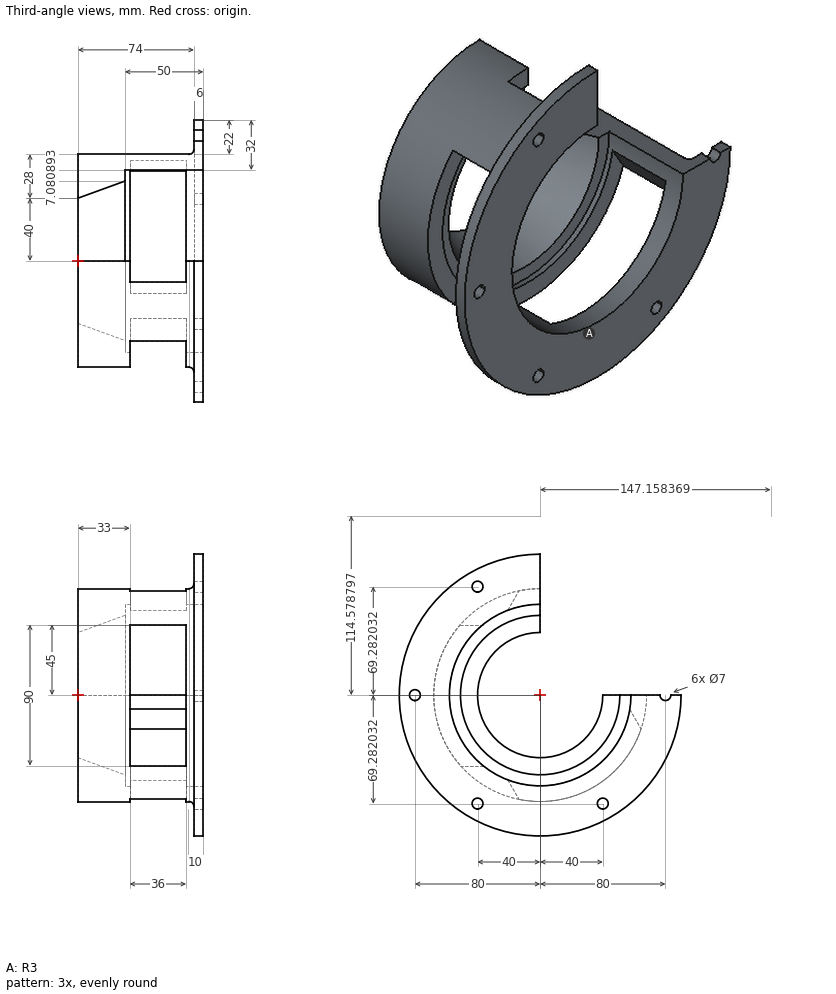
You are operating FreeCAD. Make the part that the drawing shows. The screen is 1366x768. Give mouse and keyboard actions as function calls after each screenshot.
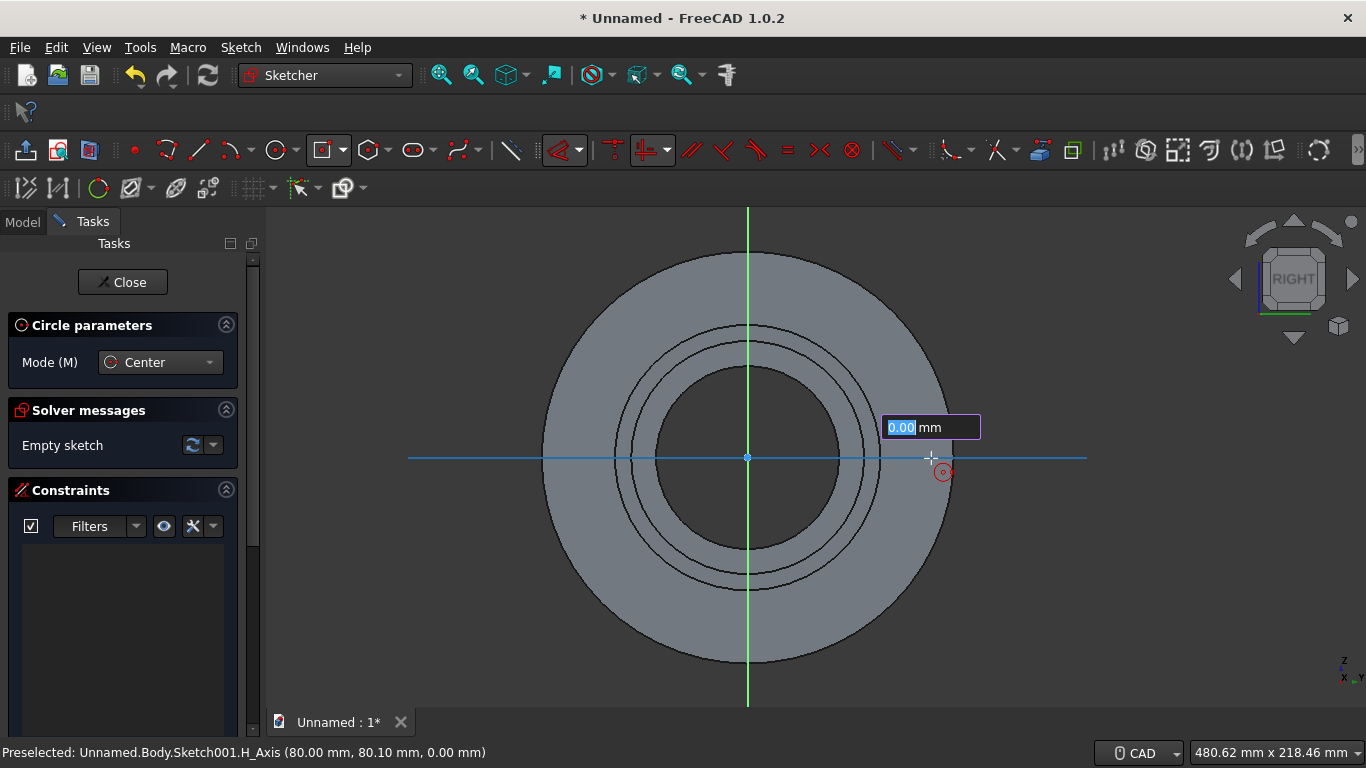
scroll(934, 450, up, 4)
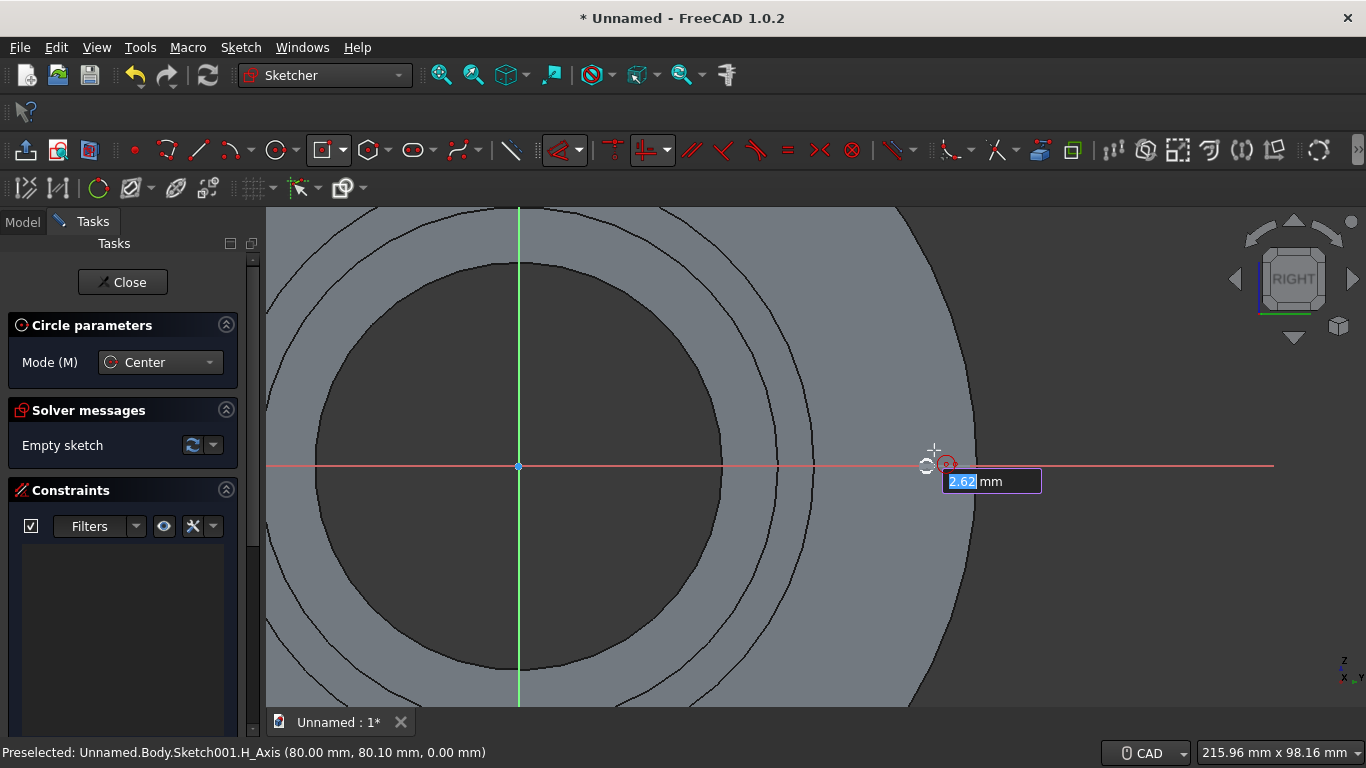
click(932, 450)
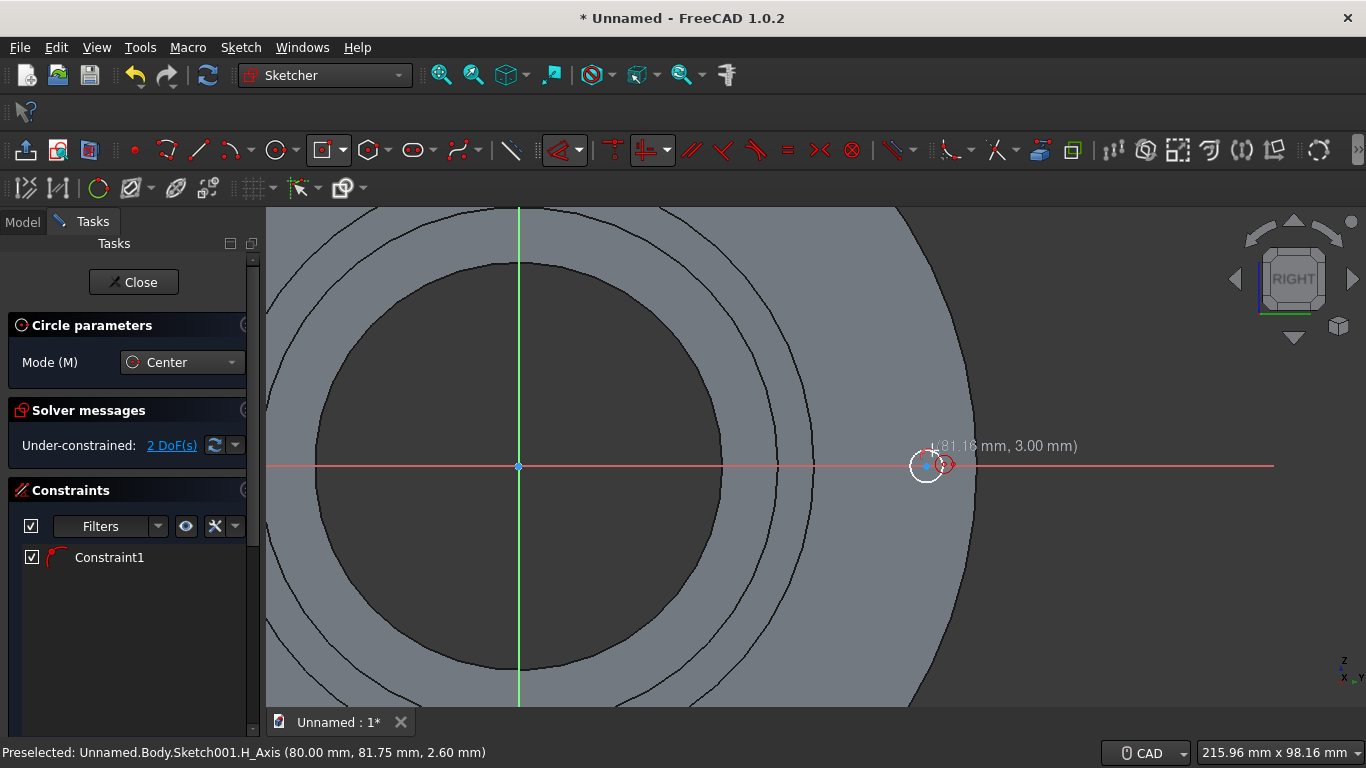
scroll(934, 449, down, 4)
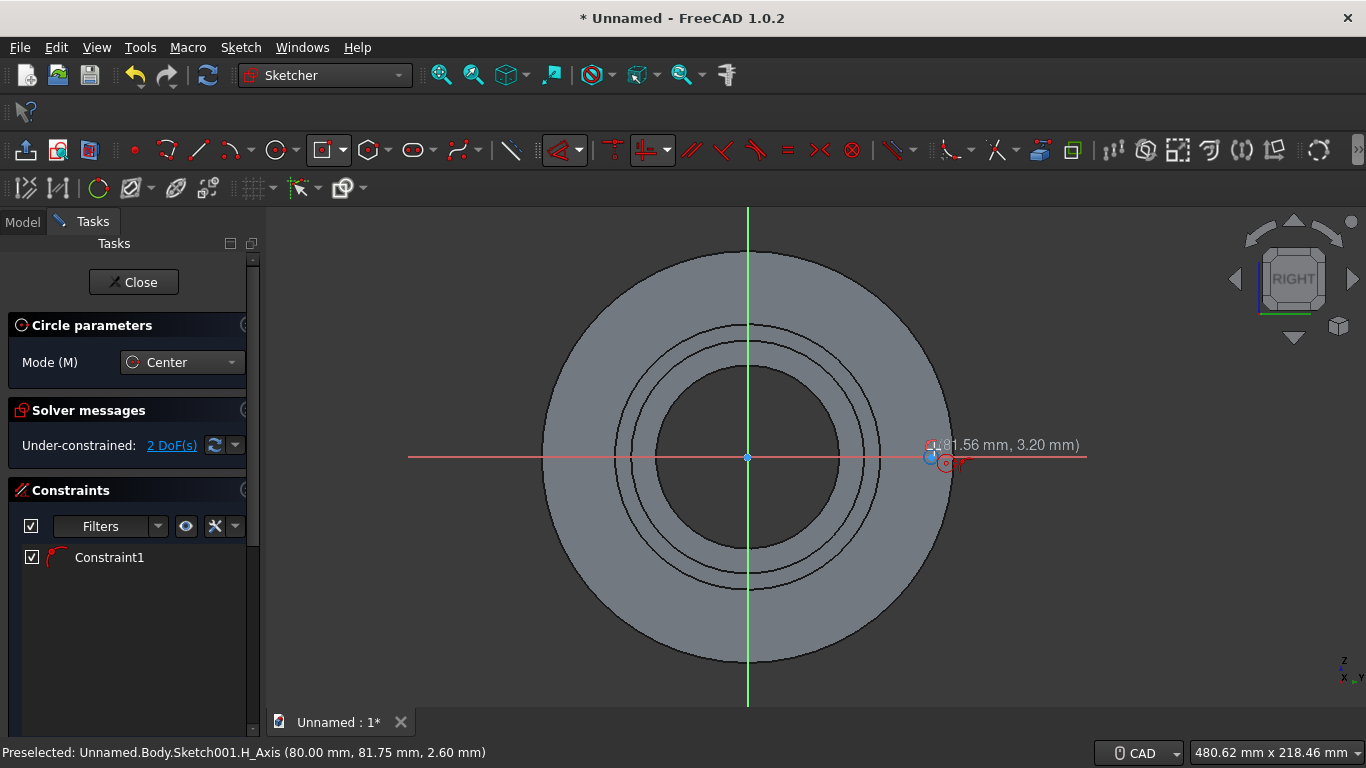
scroll(839, 616, up, 6)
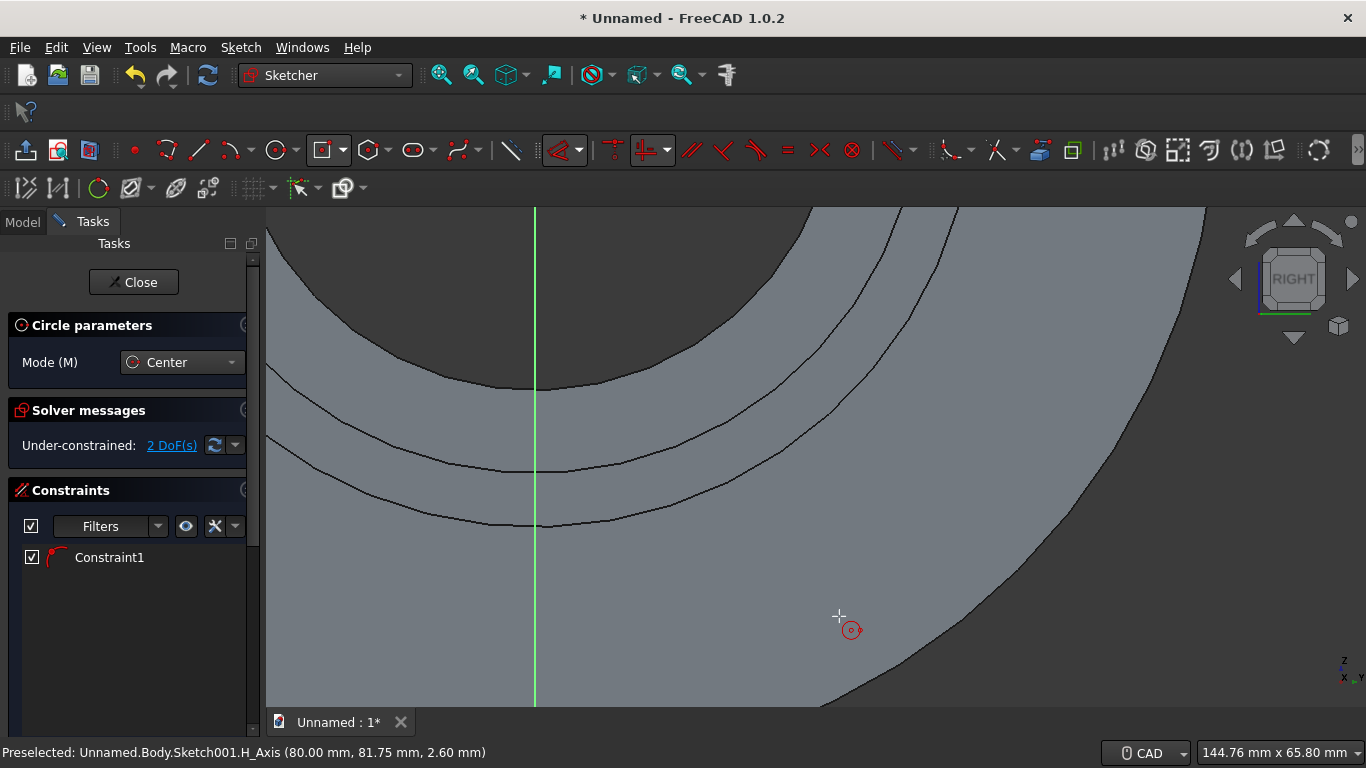
scroll(839, 617, down, 6)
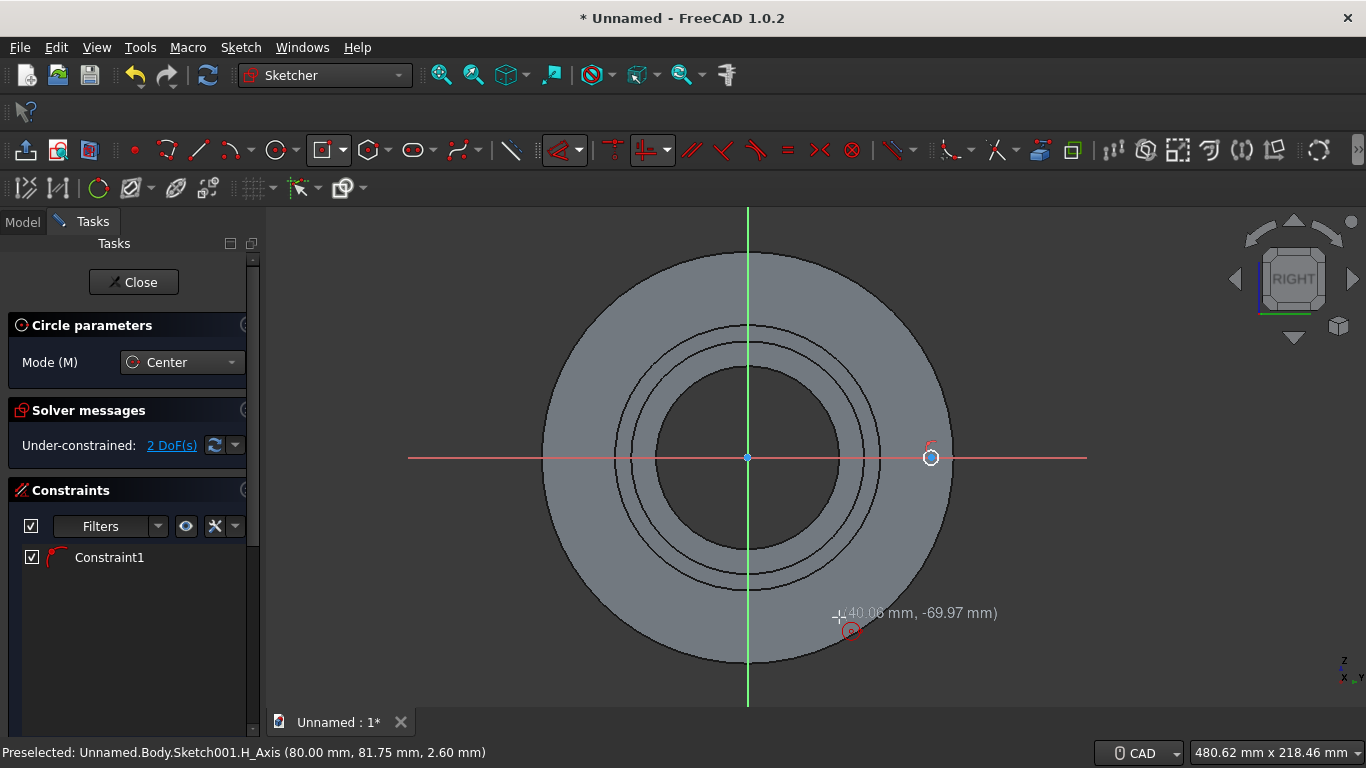
click(839, 616)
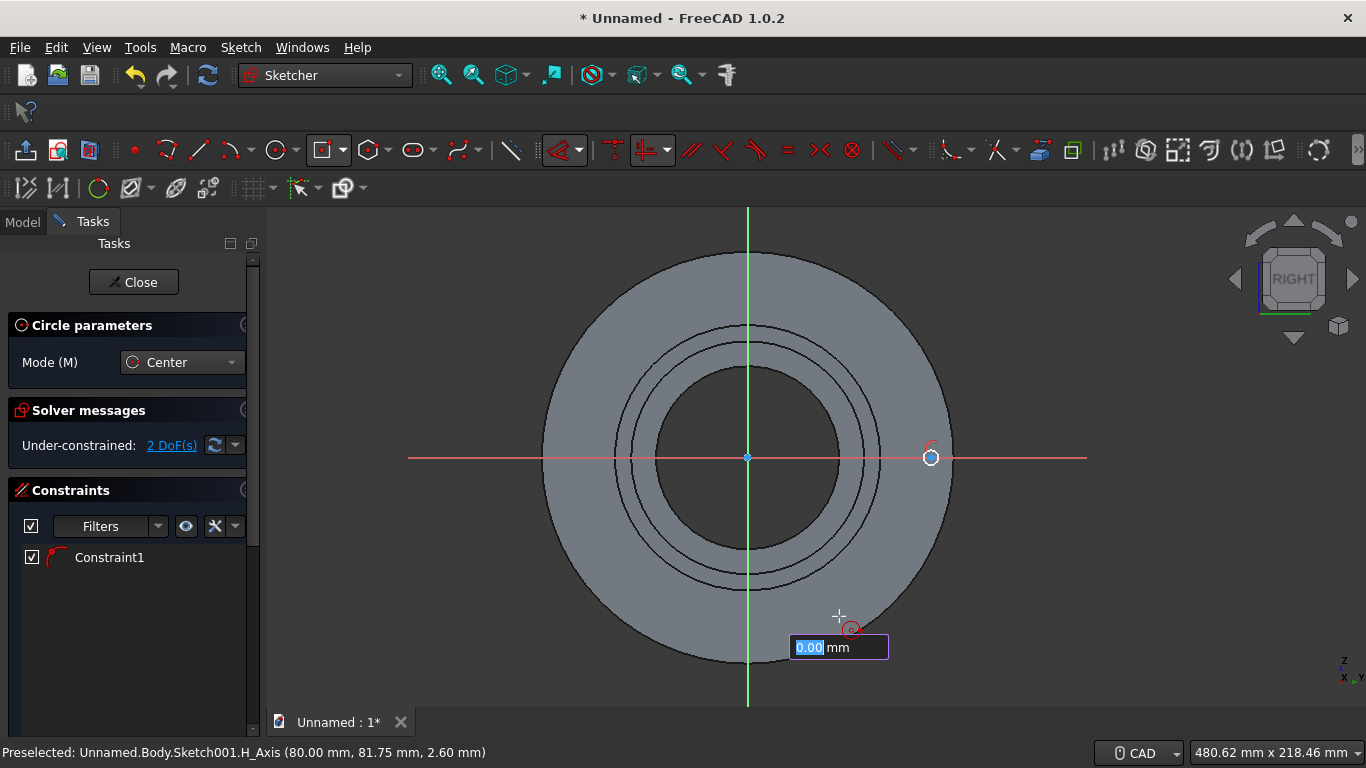
scroll(845, 611, up, 4)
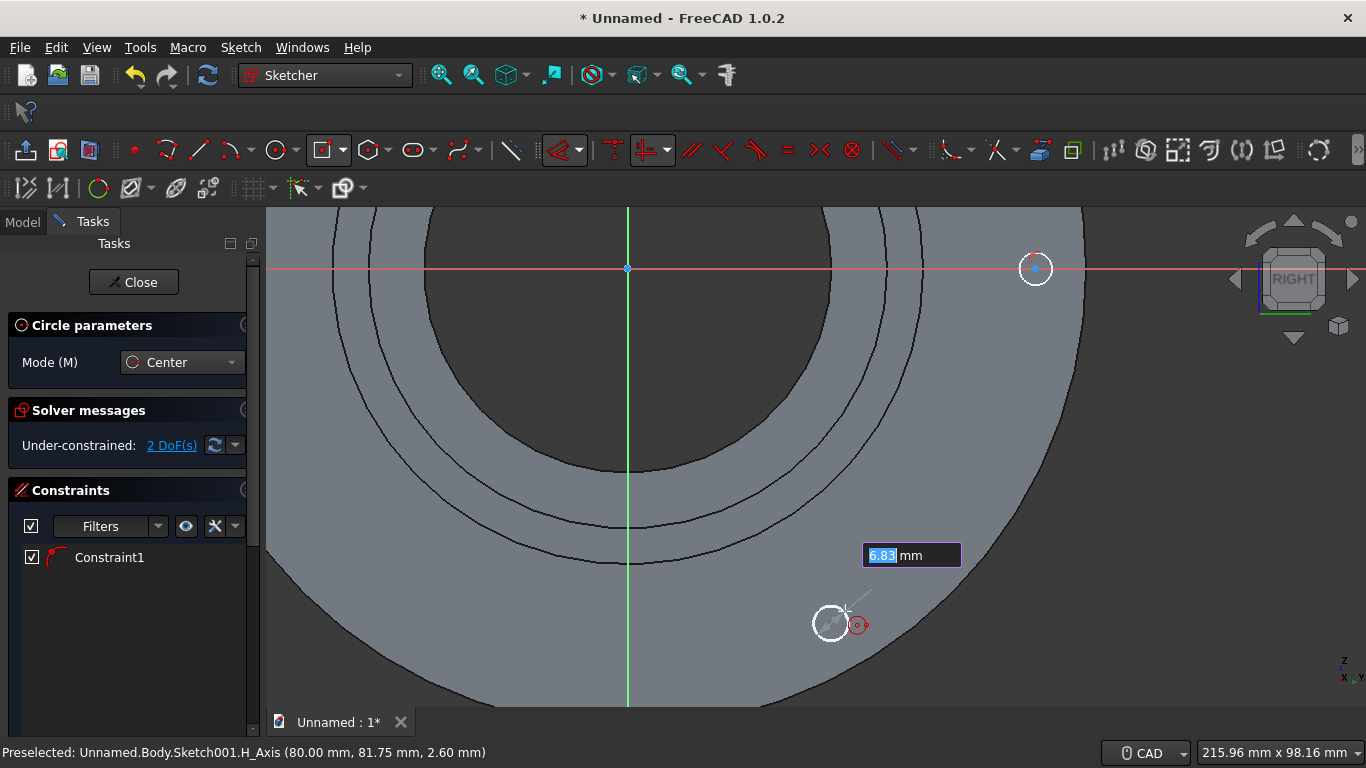
click(844, 609)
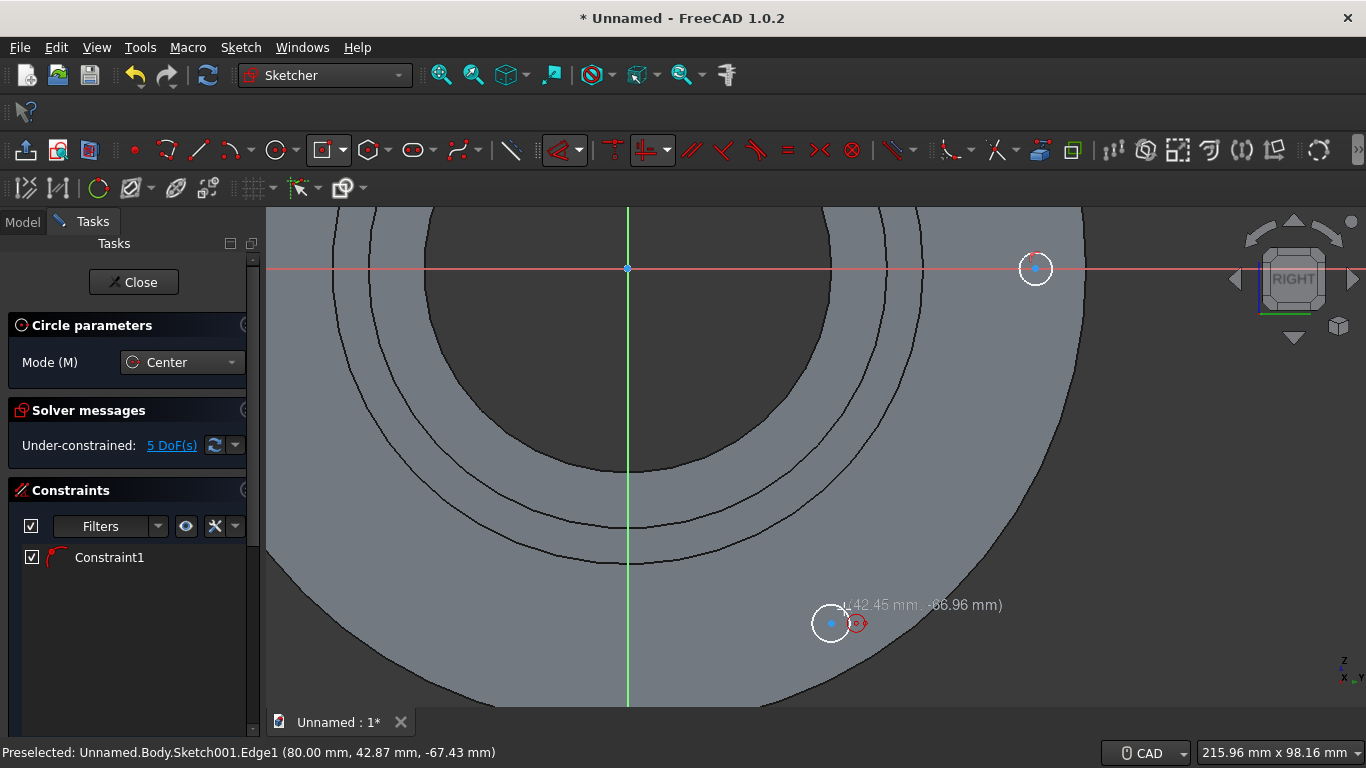
scroll(424, 622, up, 2)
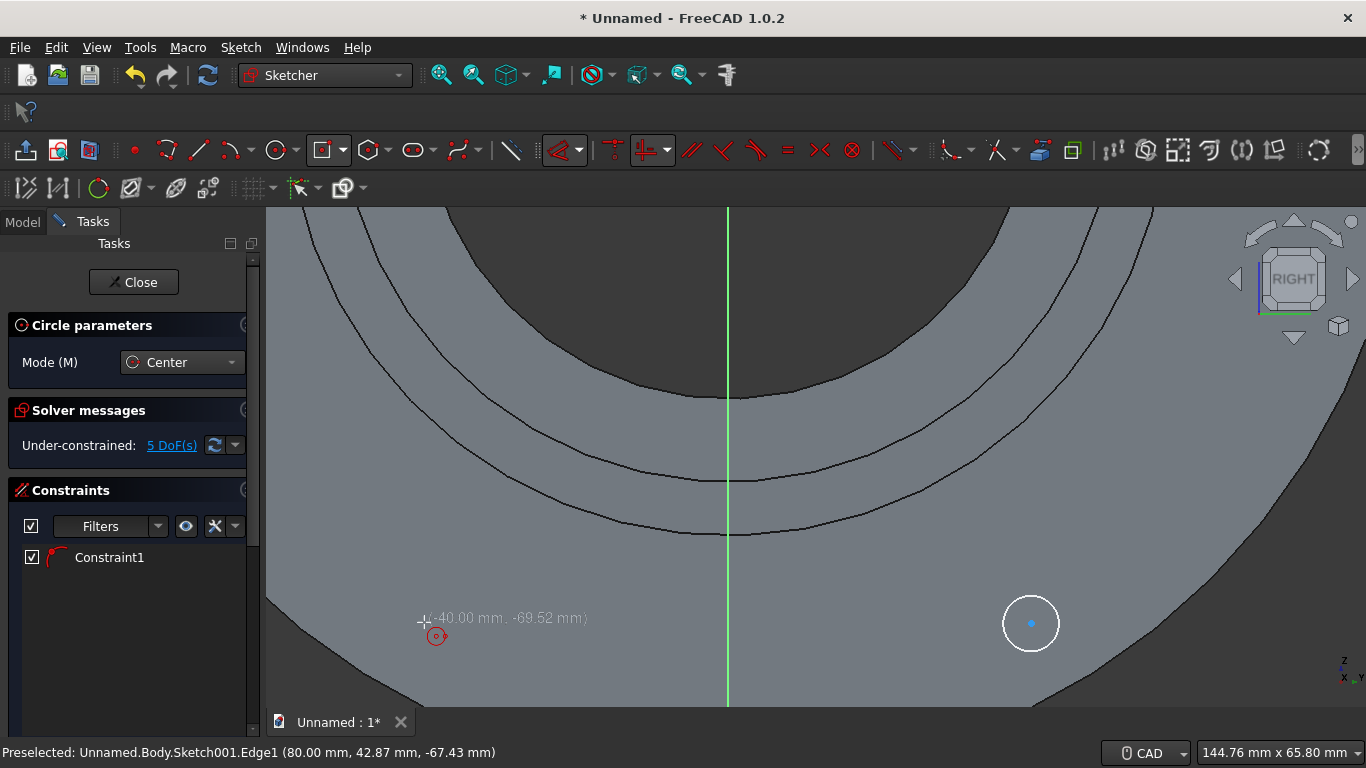
scroll(756, 613, down, 6)